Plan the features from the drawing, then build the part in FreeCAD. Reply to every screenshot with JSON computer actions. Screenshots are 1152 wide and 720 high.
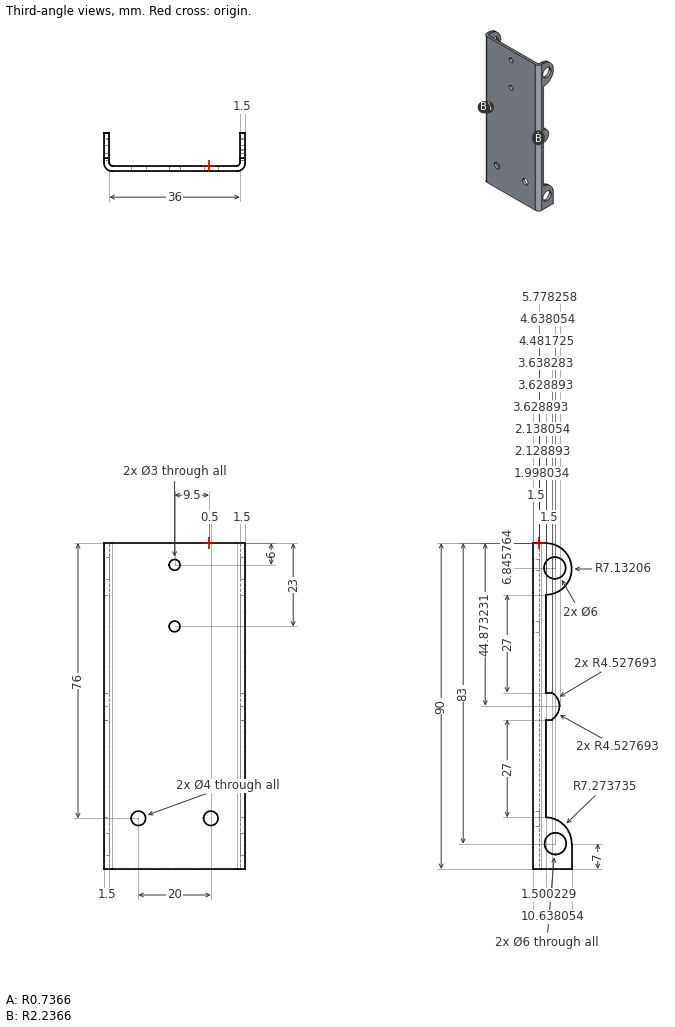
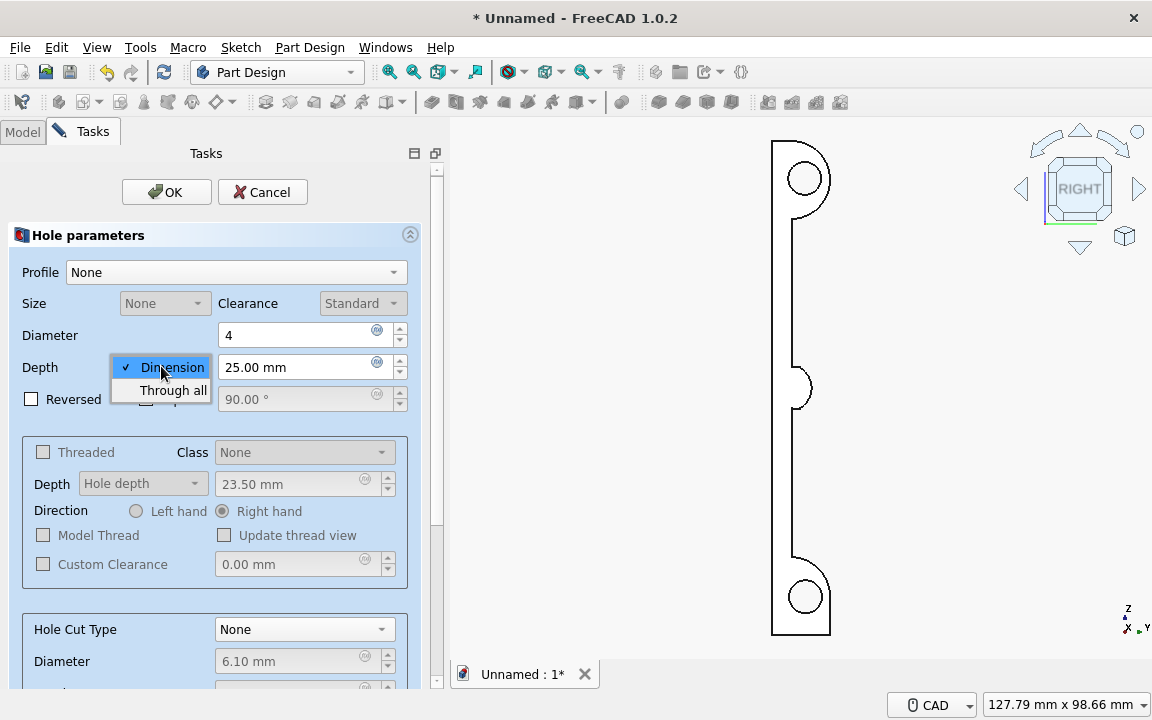
{"action": "left_click", "coordinate": [160, 390]}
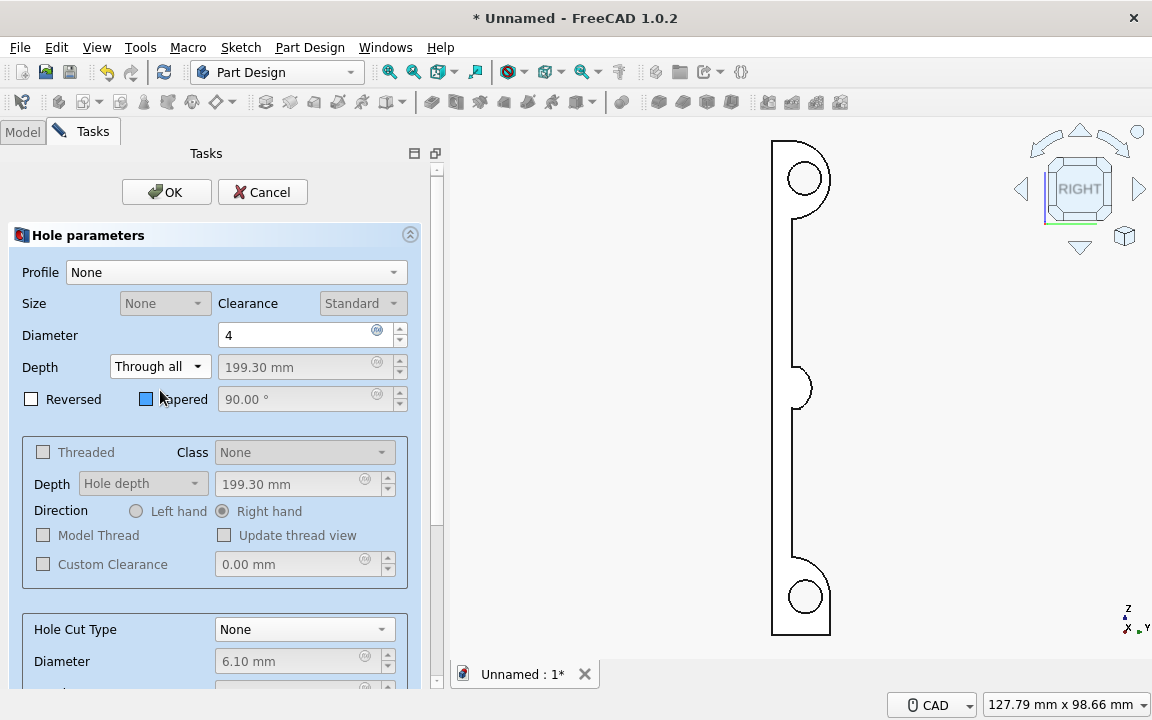
{"action": "left_click", "coordinate": [30, 399]}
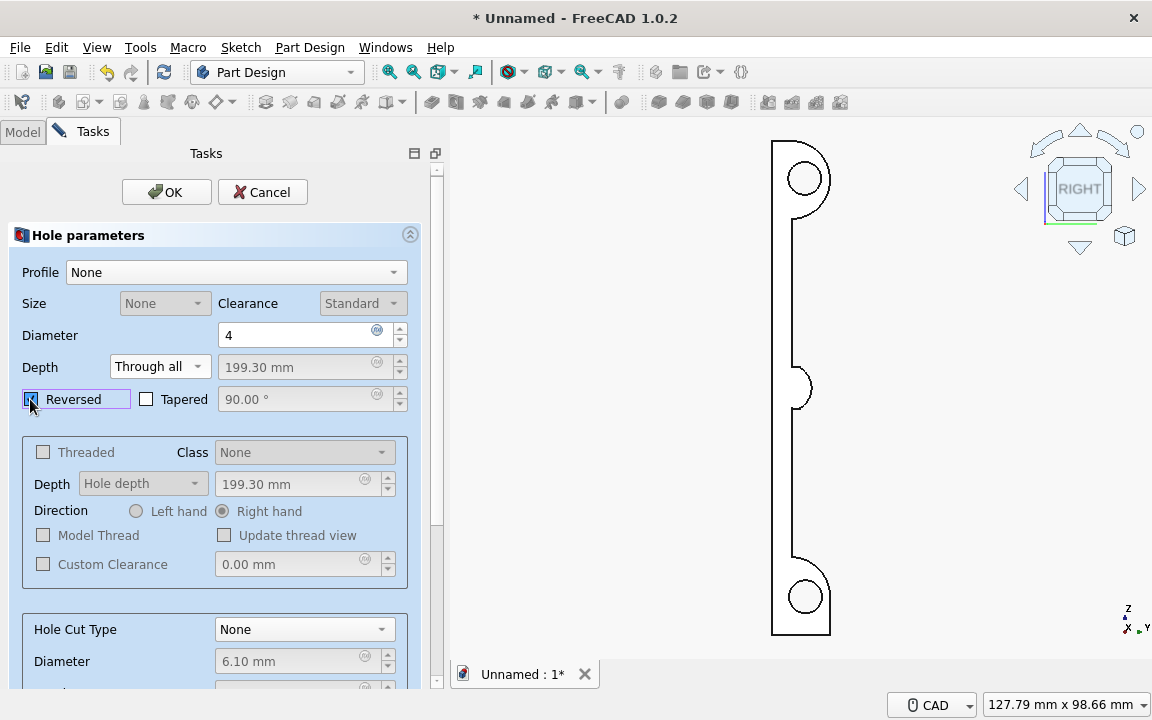
{"action": "left_click", "coordinate": [167, 192]}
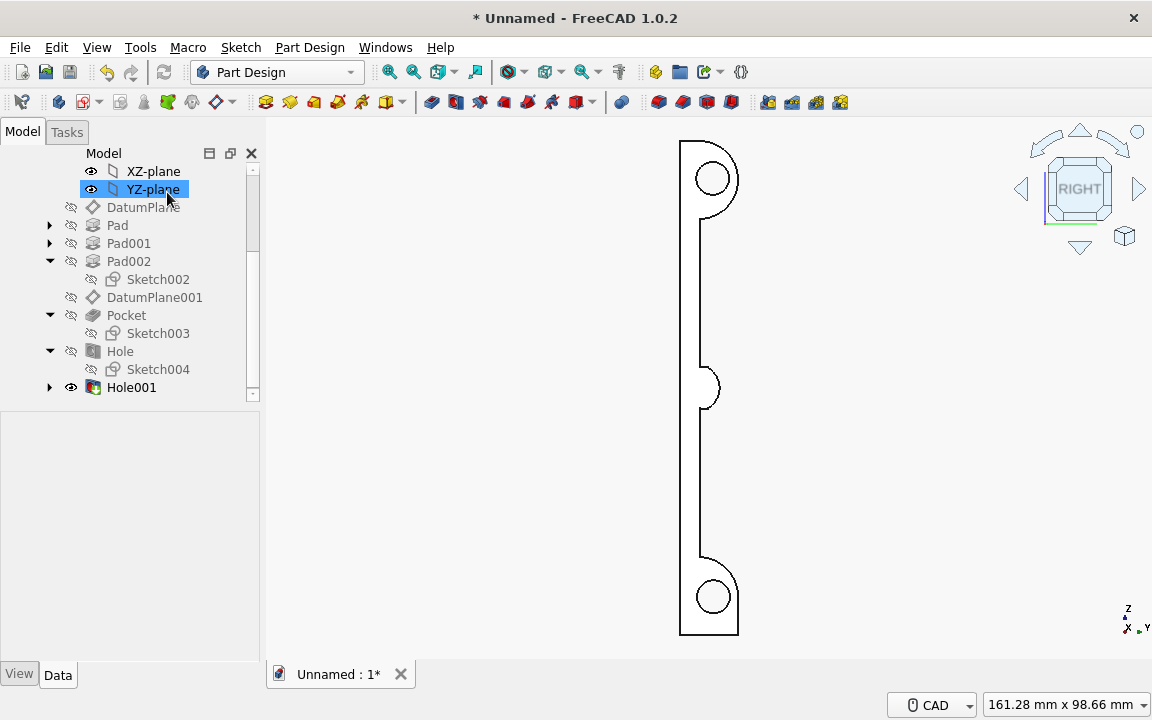
{"action": "left_click", "coordinate": [84, 102]}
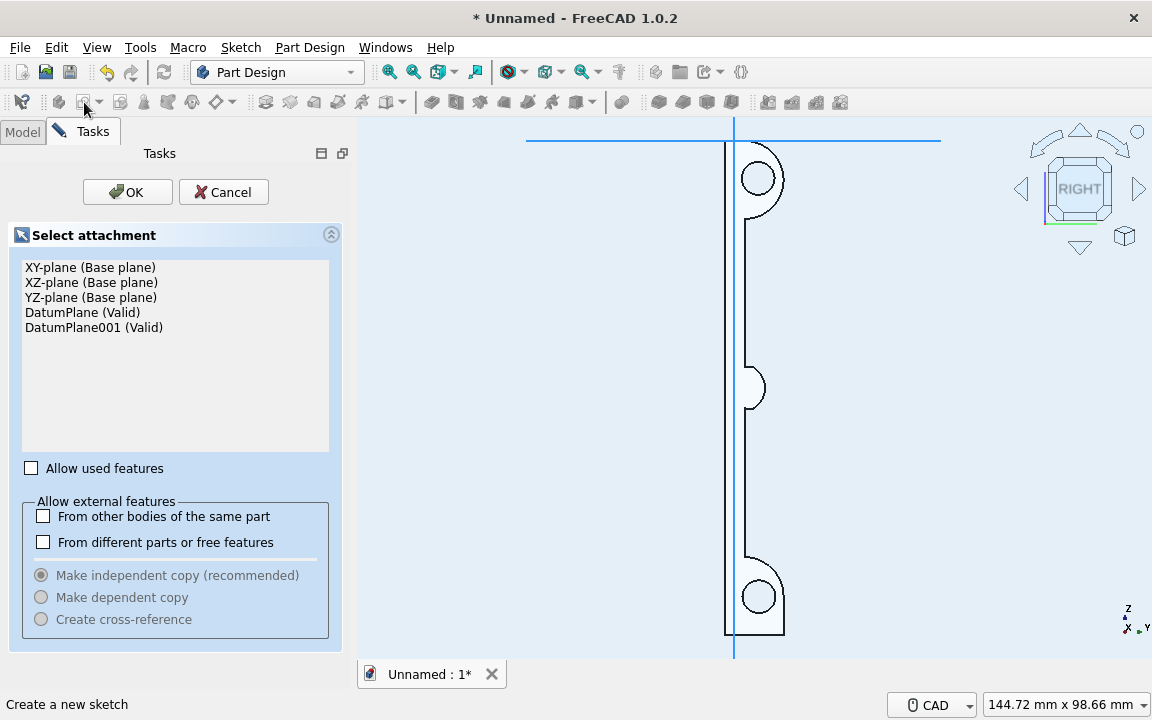
{"action": "left_click", "coordinate": [82, 282]}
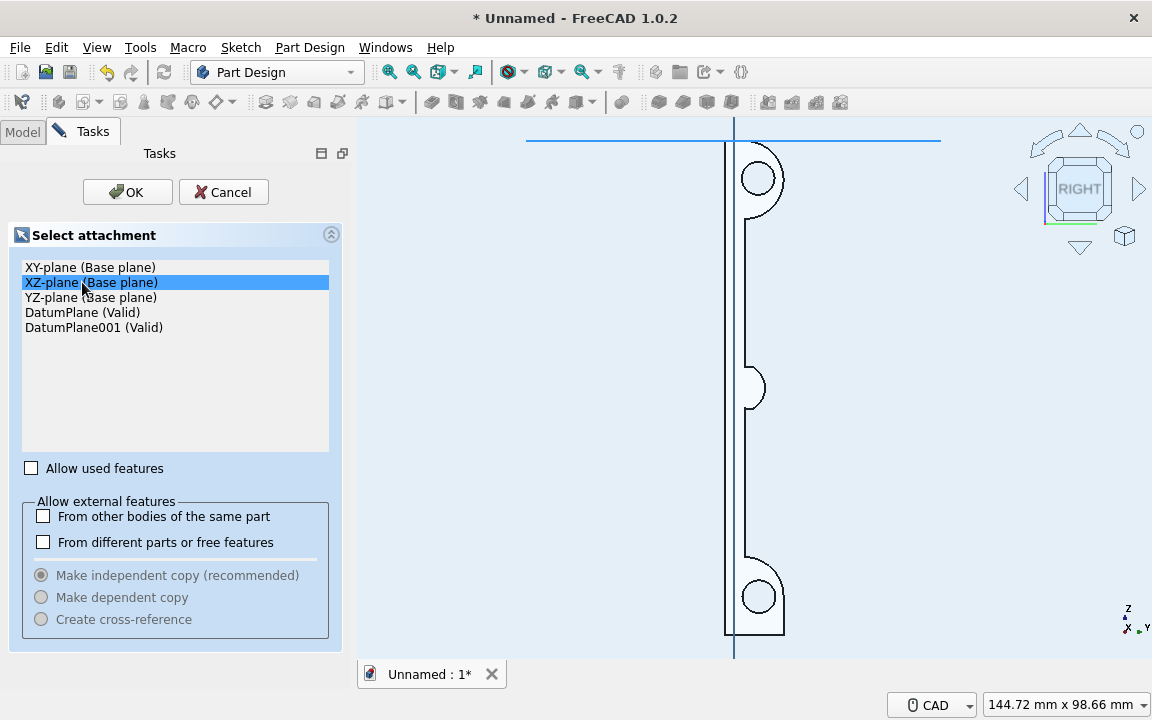
{"action": "left_click", "coordinate": [128, 192]}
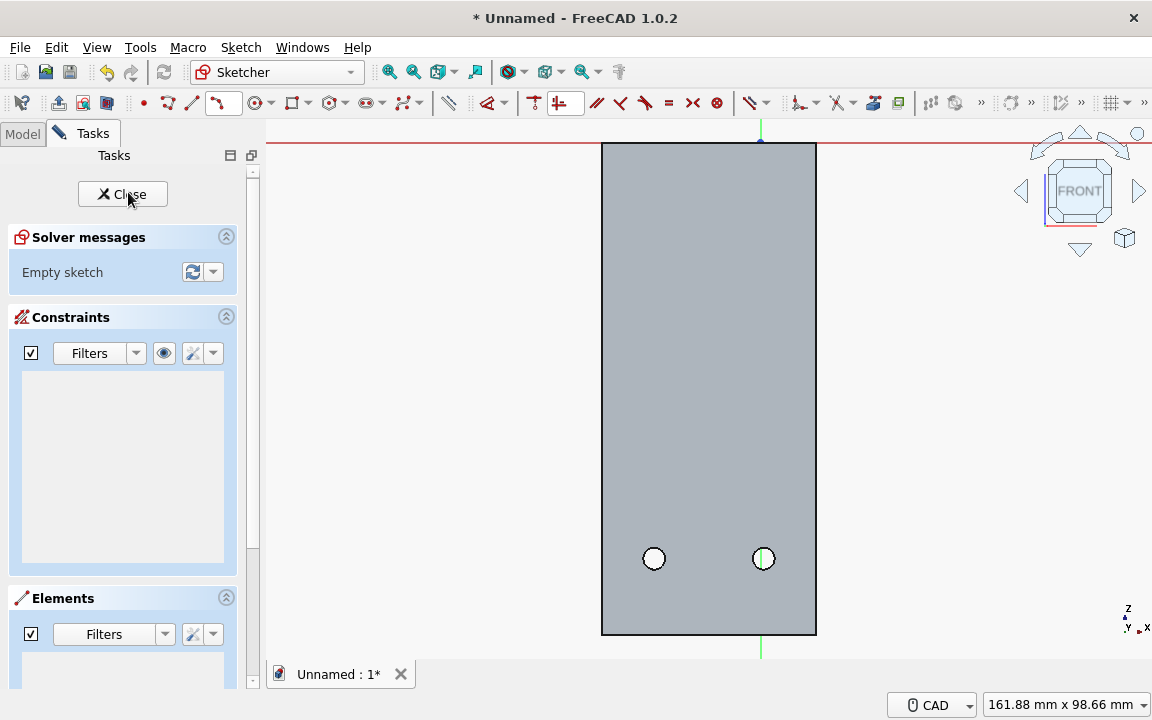
{"action": "left_click", "coordinate": [108, 104]}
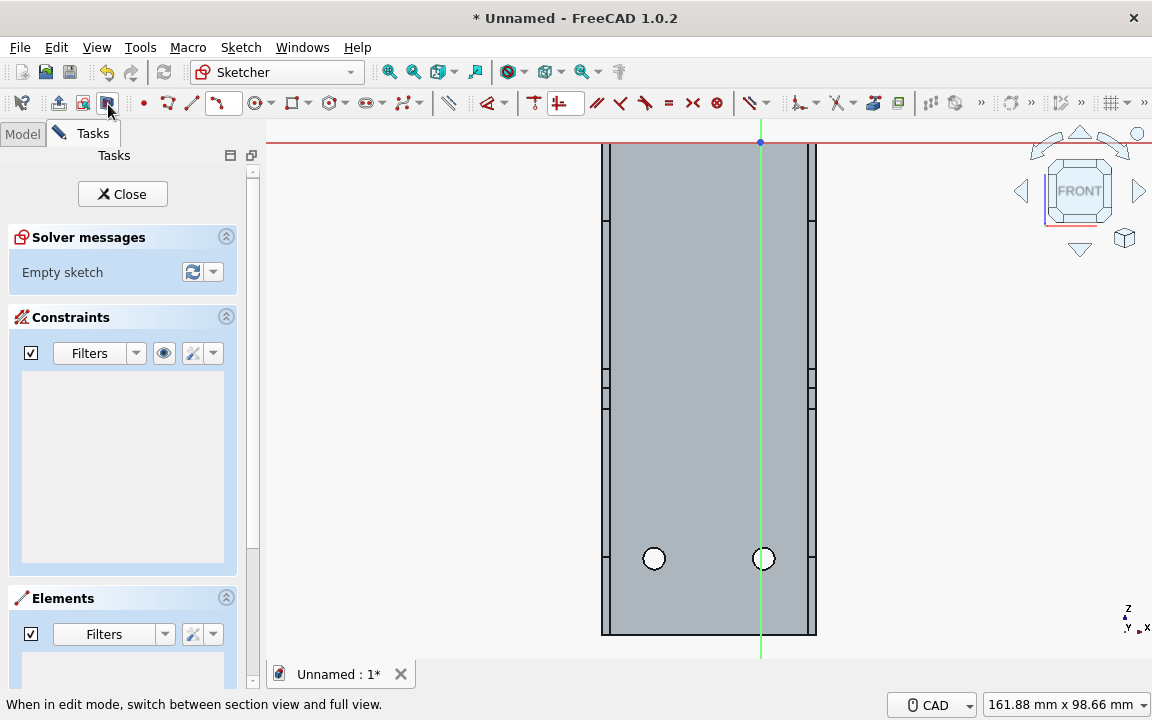
{"action": "scroll", "coordinate": [640, 389], "scroll_direction": "down", "scroll_amount": 5}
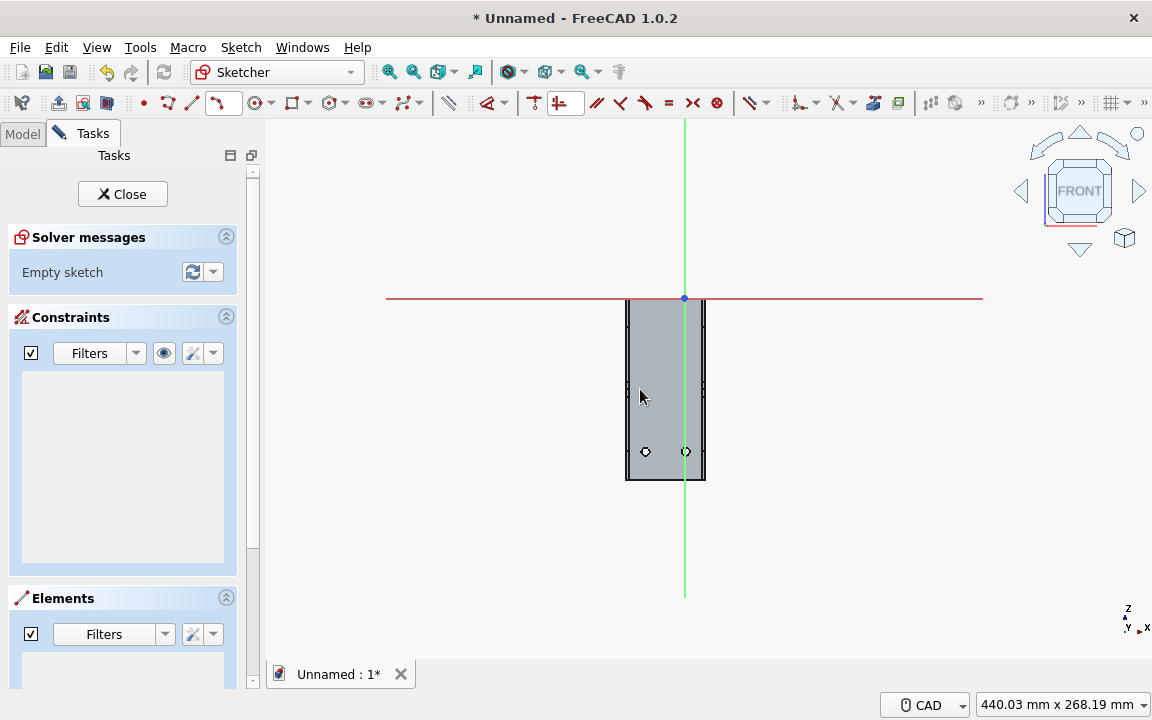
{"action": "scroll", "coordinate": [679, 313], "scroll_direction": "up", "scroll_amount": 10}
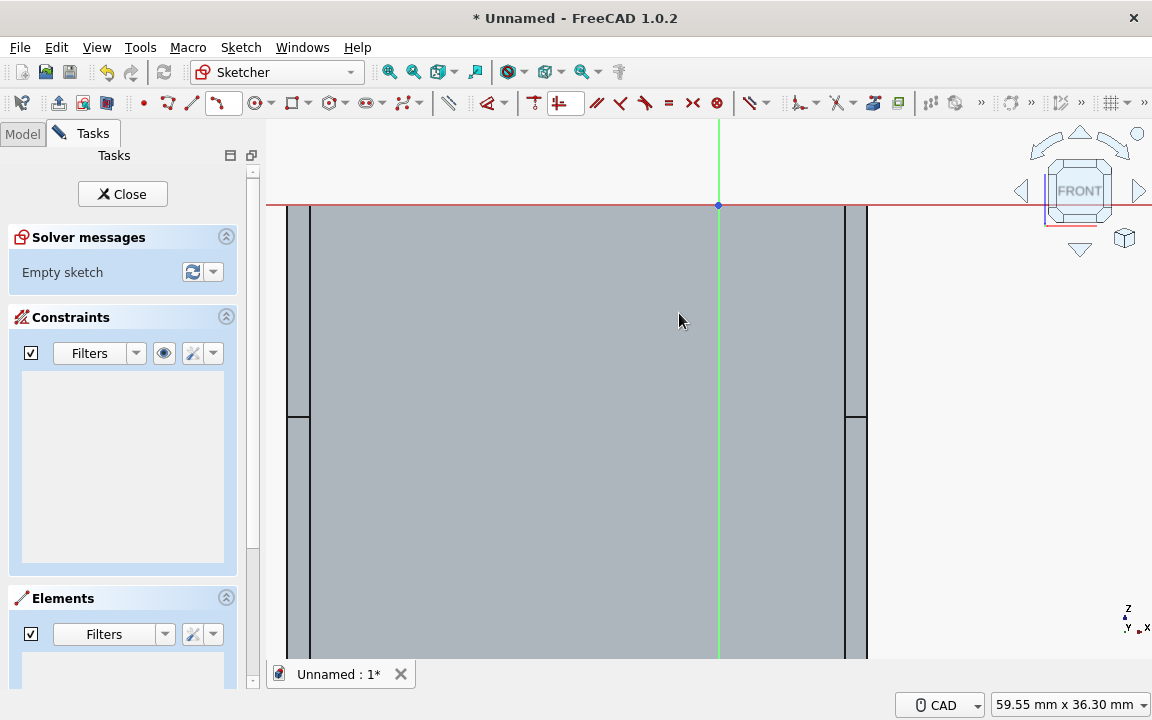
{"action": "left_click", "coordinate": [256, 104]}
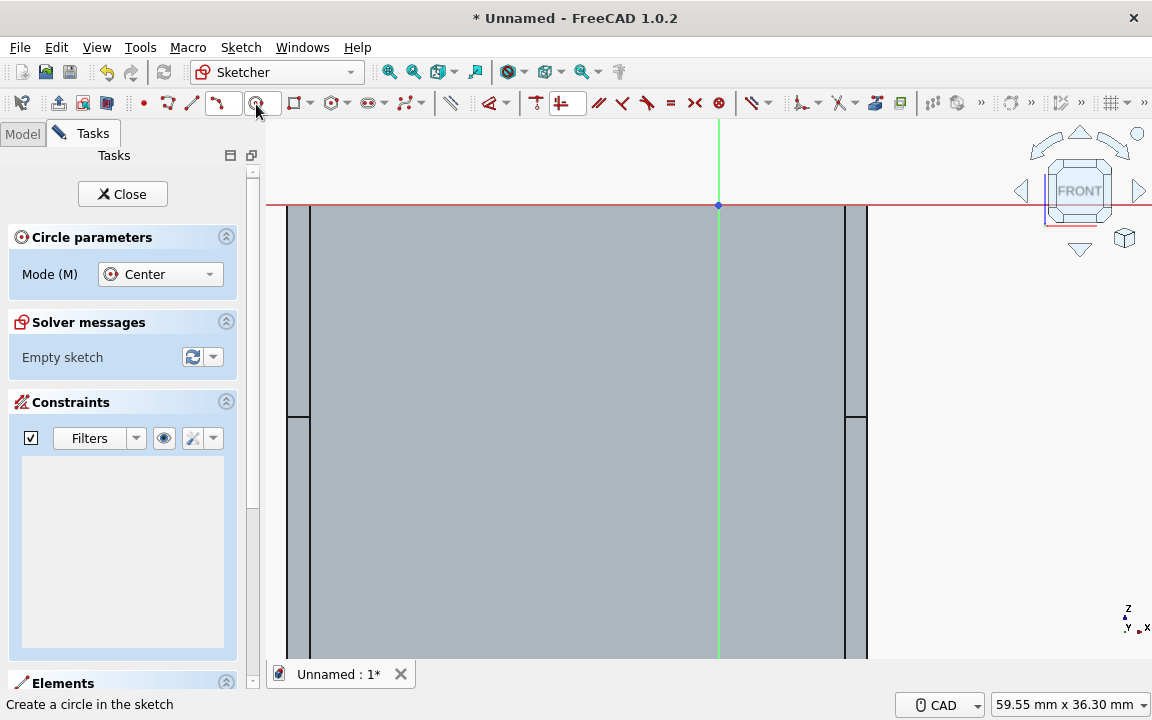
{"action": "left_click", "coordinate": [577, 294]}
{"action": "left_click", "coordinate": [593, 279]}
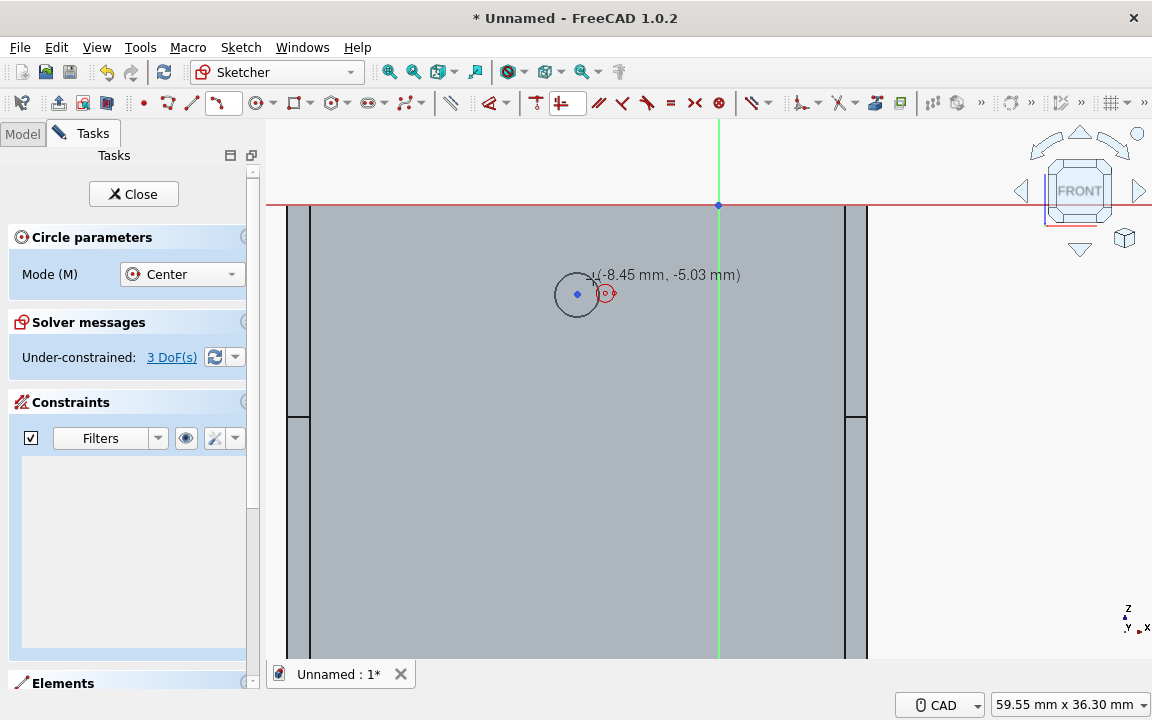
{"action": "left_click", "coordinate": [577, 547]}
{"action": "left_click", "coordinate": [593, 532]}
{"action": "key", "text": "Escape"}